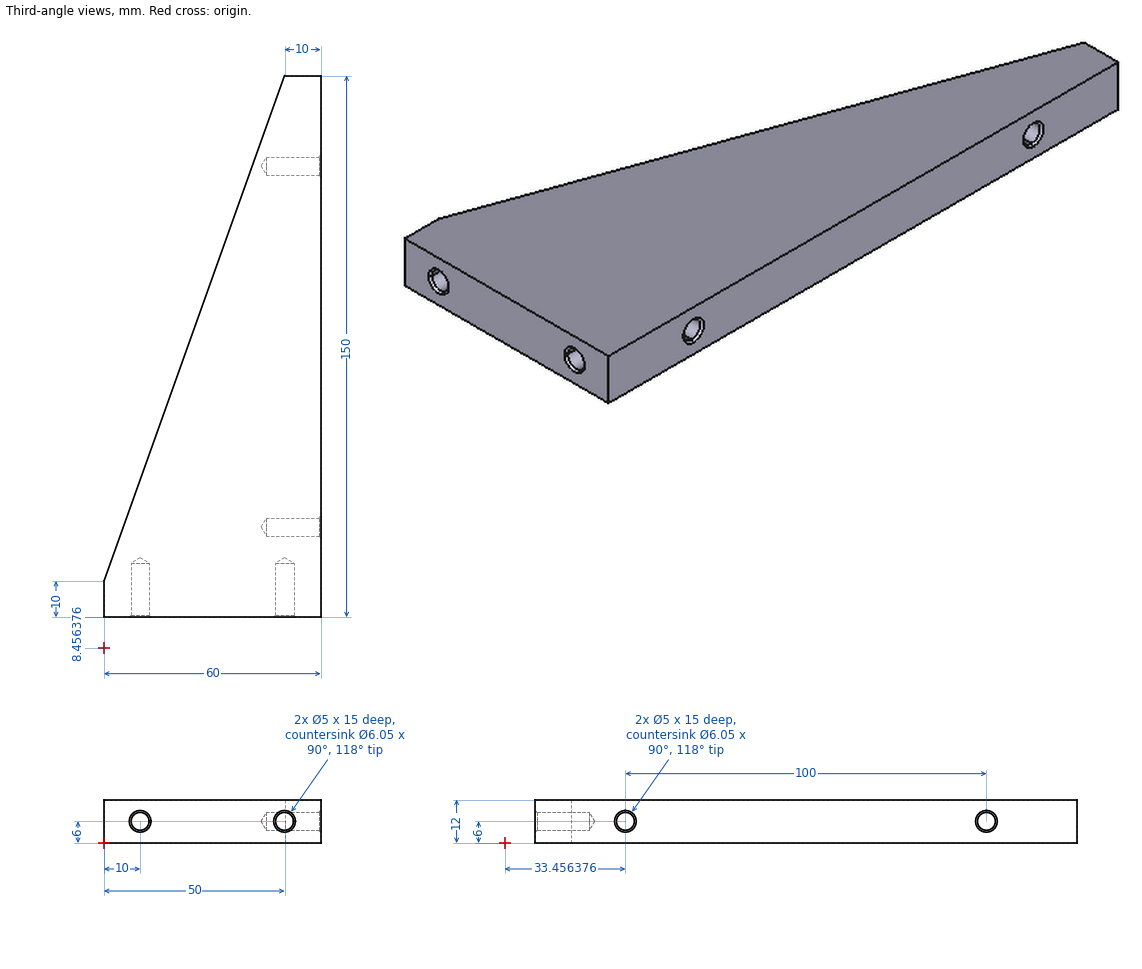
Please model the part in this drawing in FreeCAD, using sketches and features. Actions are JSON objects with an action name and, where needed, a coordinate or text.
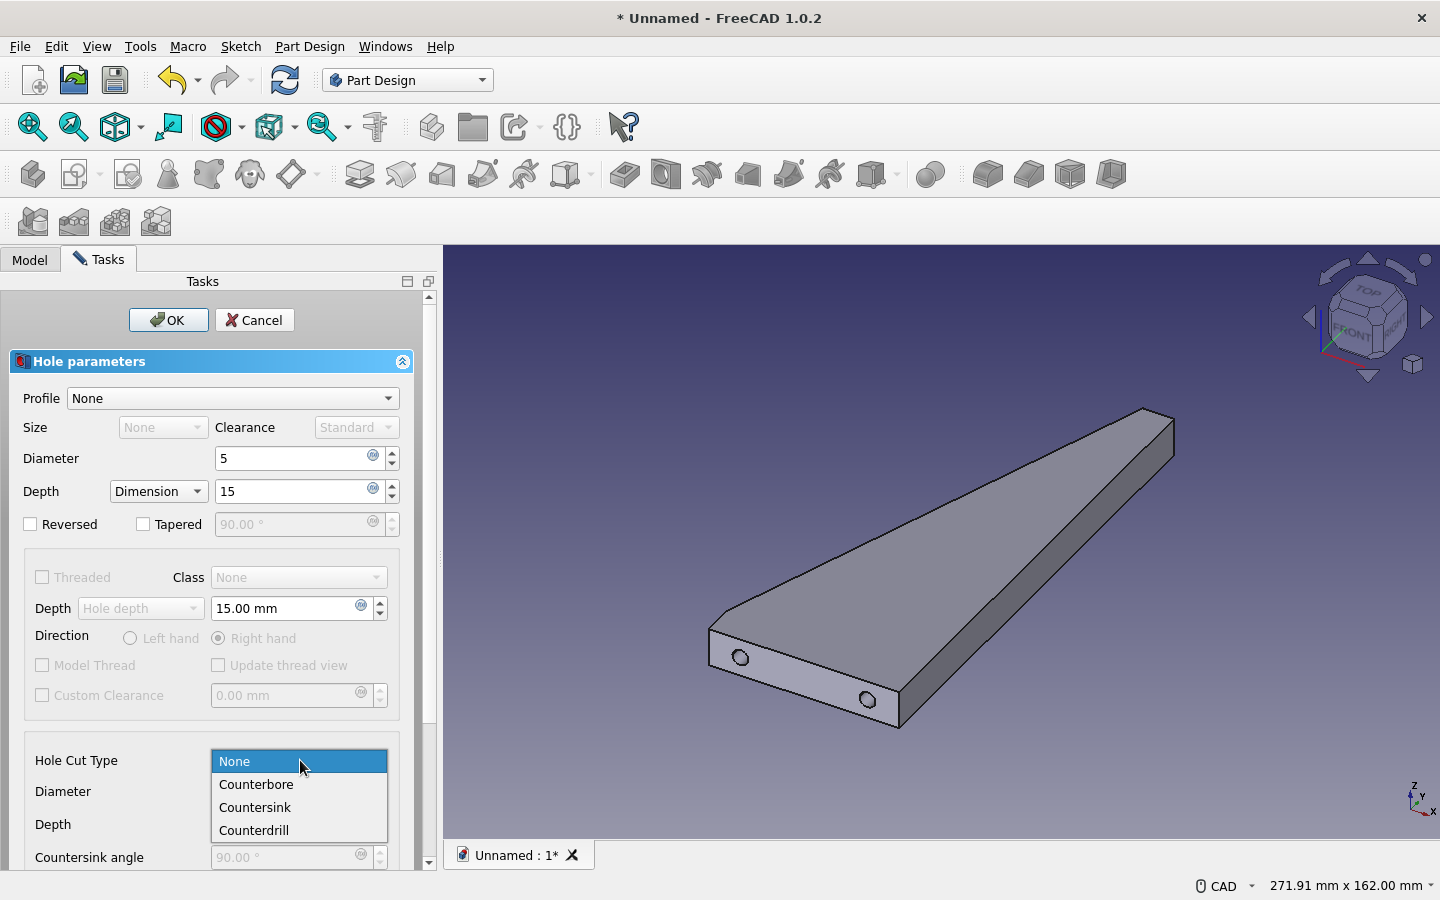
{"action": "left_click", "coordinate": [298, 808]}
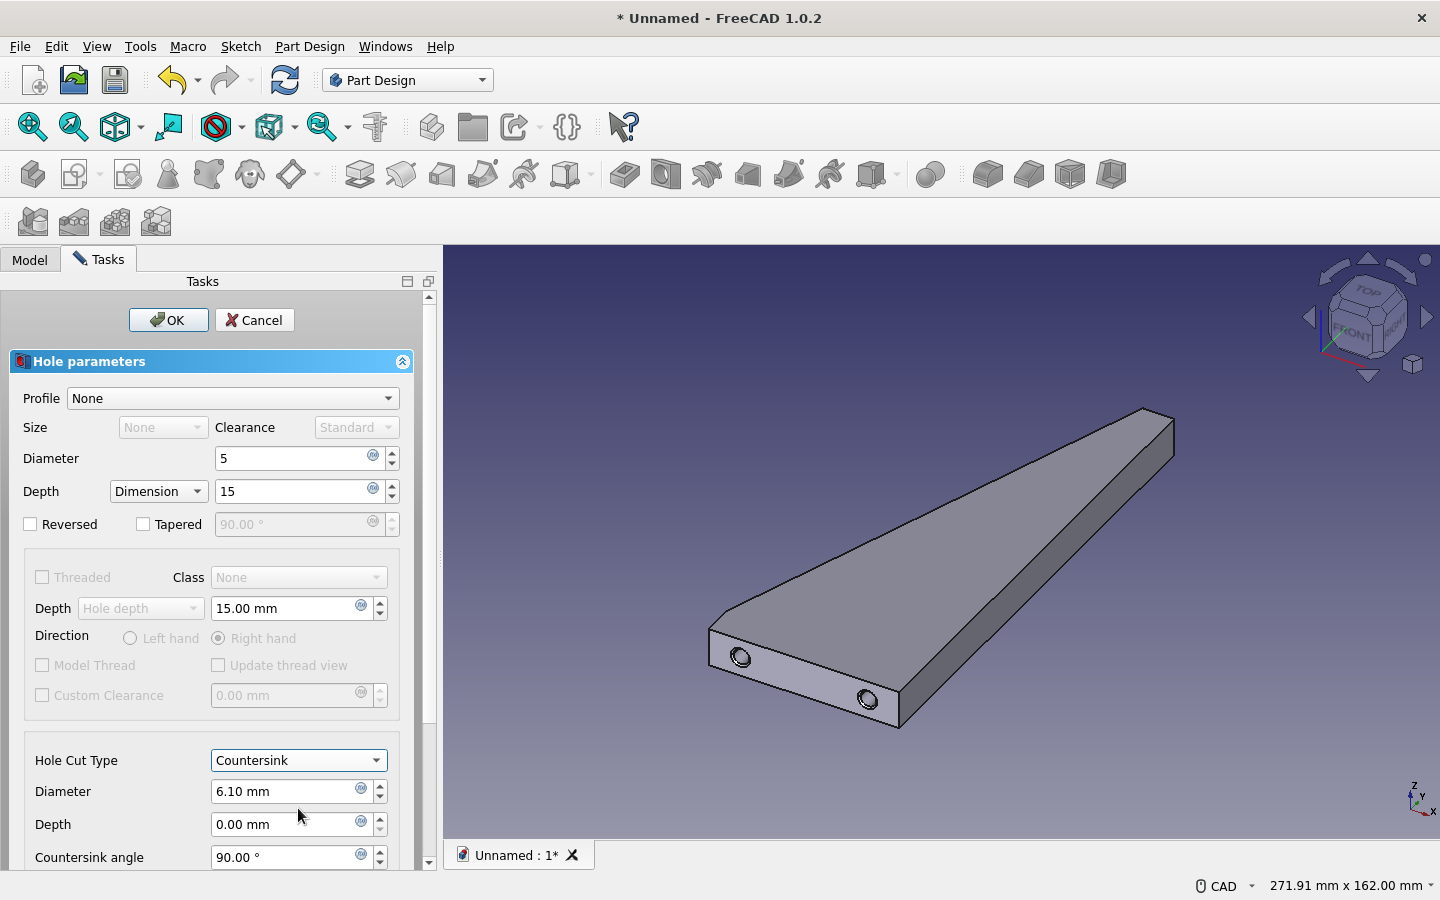
{"action": "triple_click", "coordinate": [292, 792]}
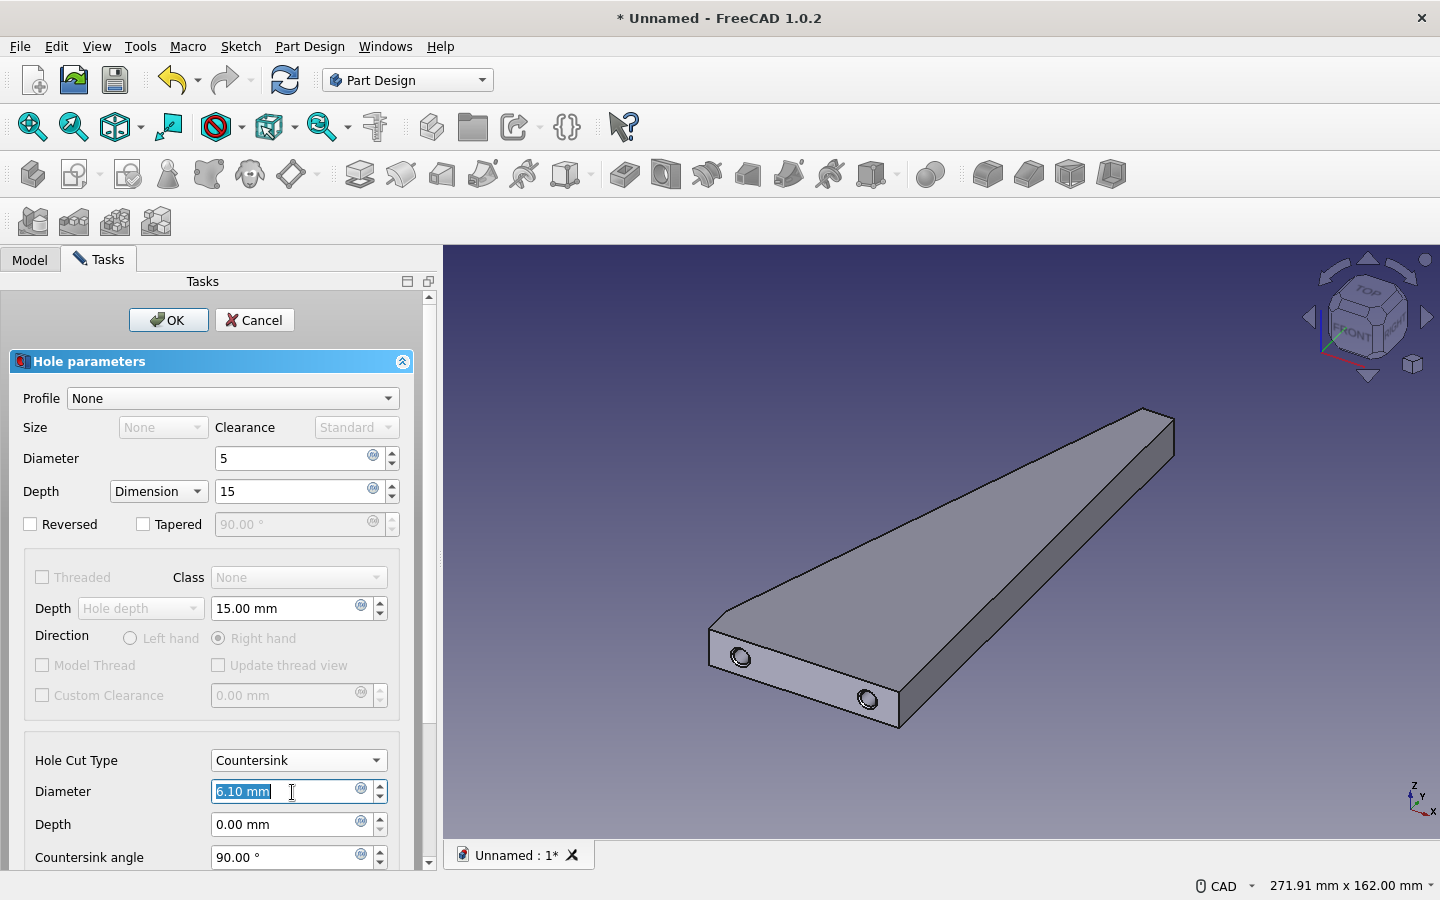
{"action": "type", "text": "6.05"}
{"action": "key", "text": "Tab"}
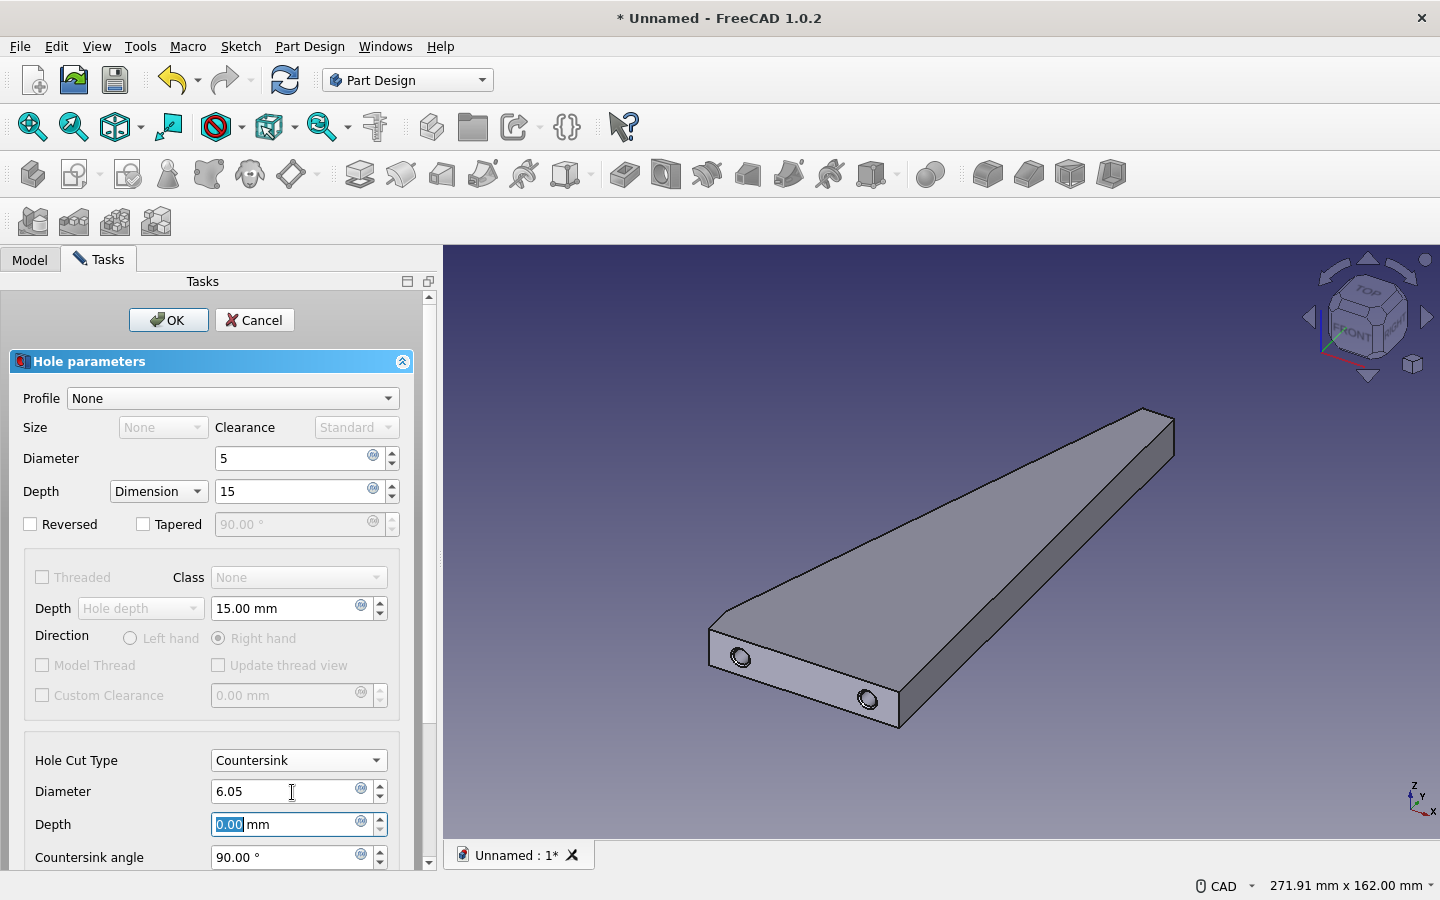
{"action": "left_click", "coordinate": [169, 320]}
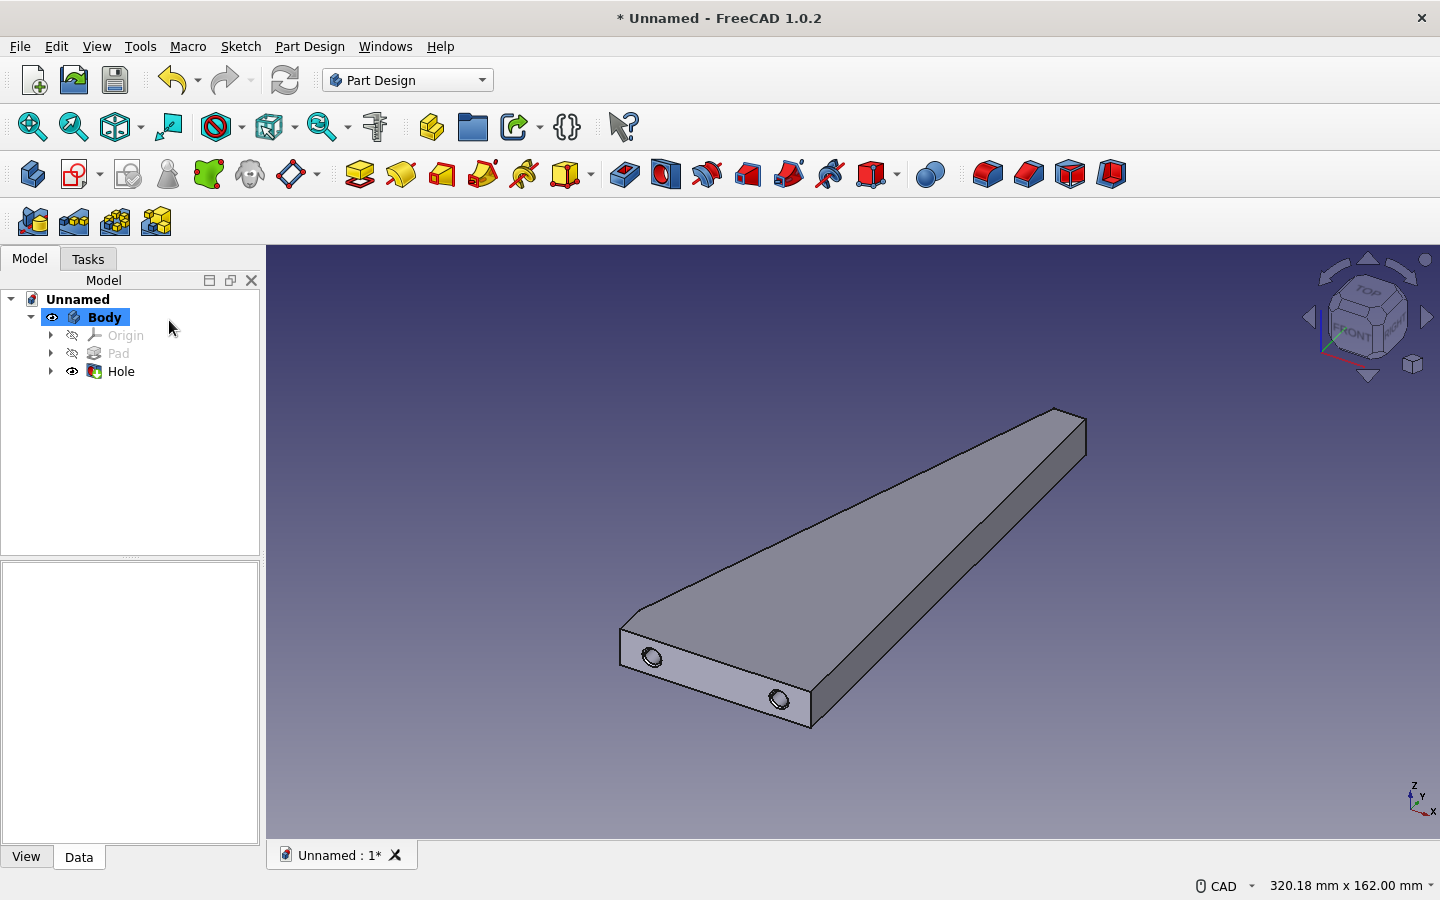
{"action": "left_click", "coordinate": [1066, 455]}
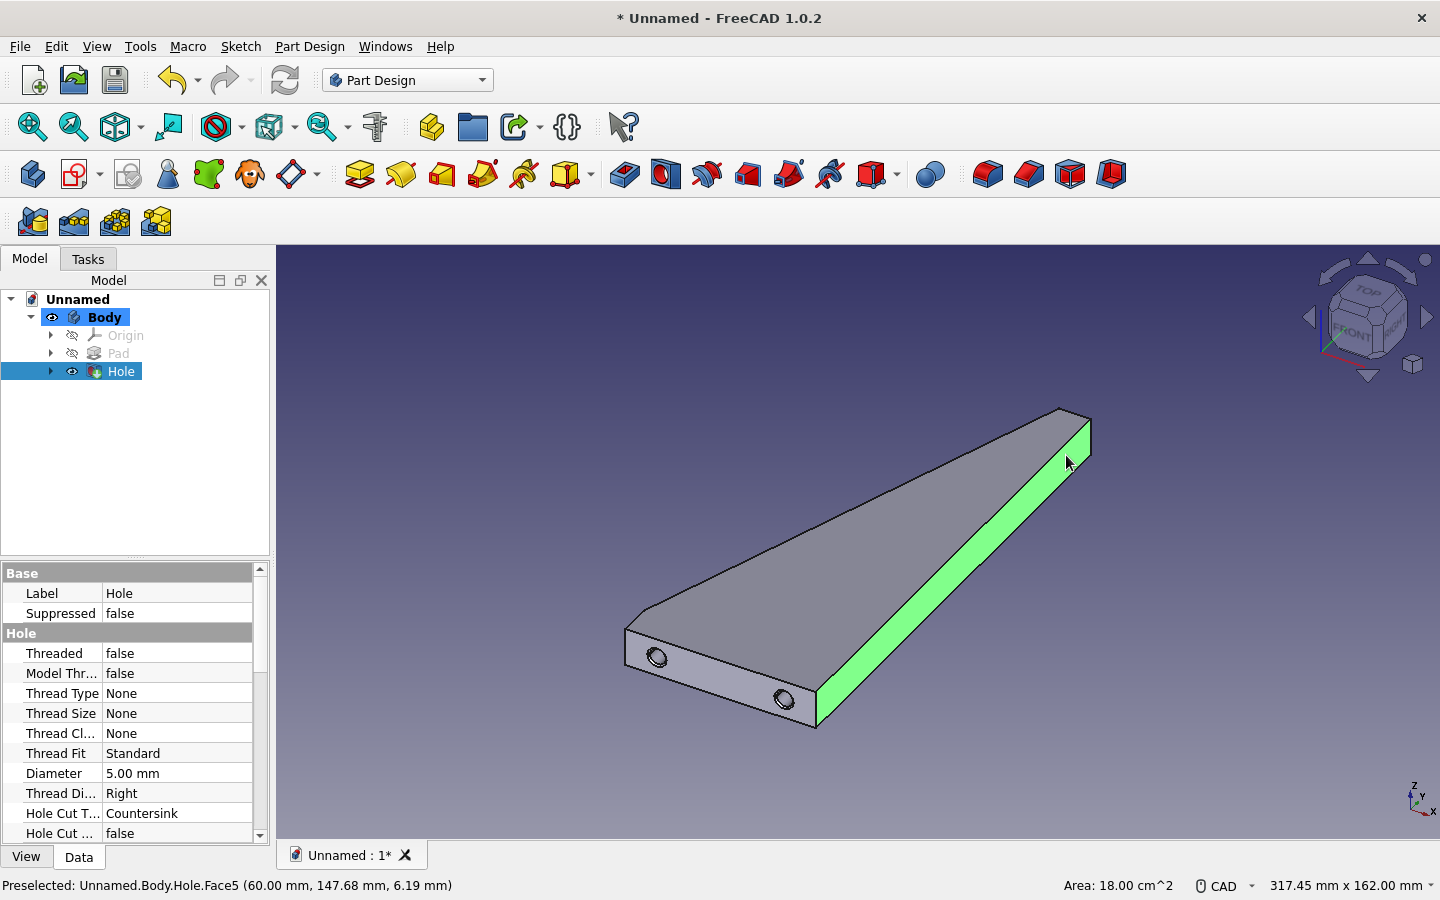
{"action": "left_click", "coordinate": [74, 174]}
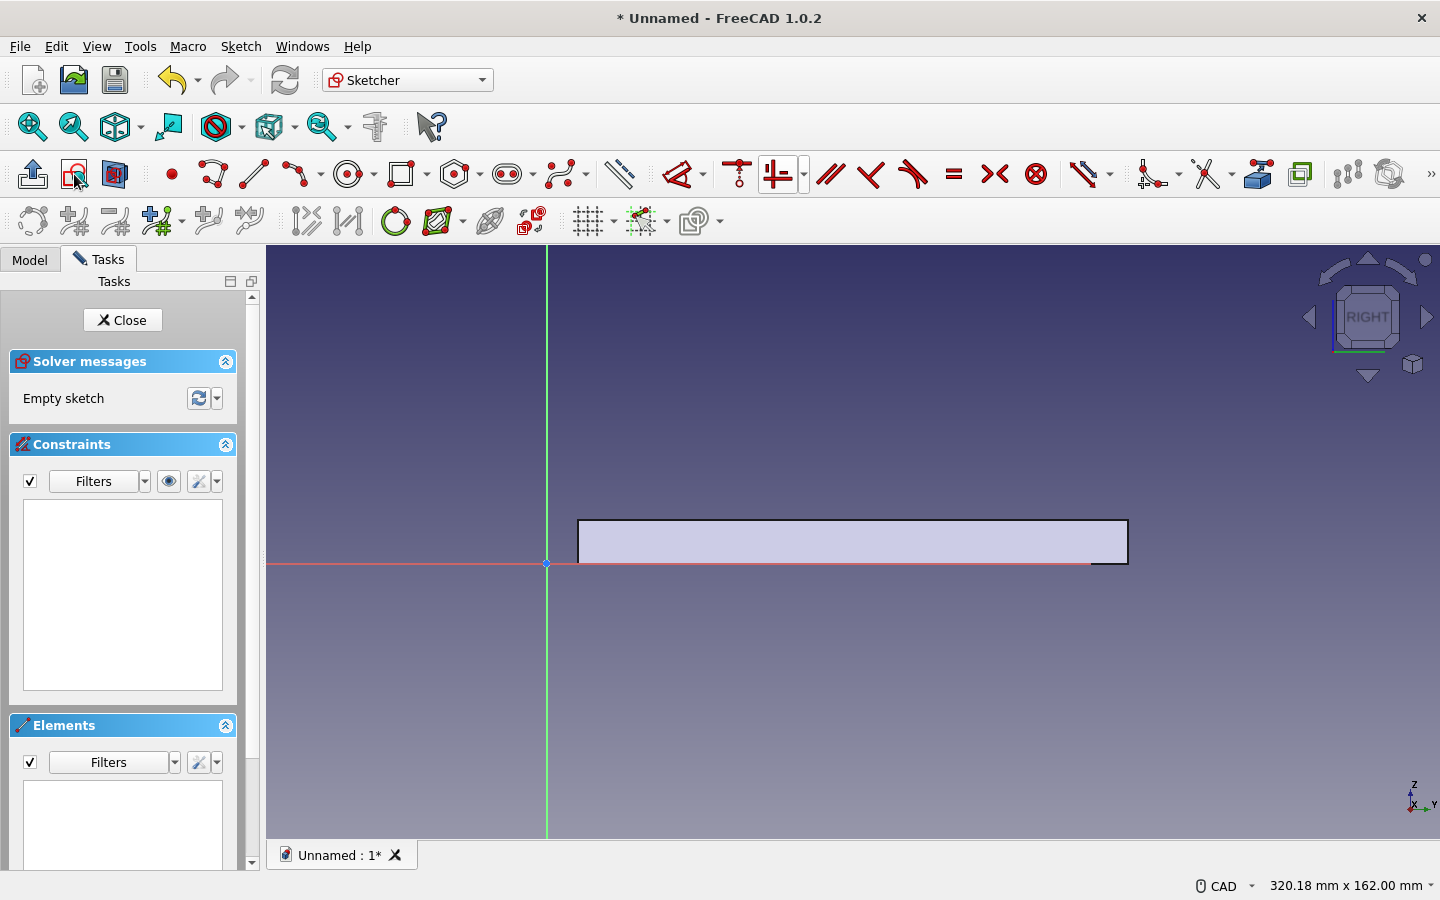
{"action": "scroll", "coordinate": [820, 561], "scroll_direction": "up", "scroll_amount": 2}